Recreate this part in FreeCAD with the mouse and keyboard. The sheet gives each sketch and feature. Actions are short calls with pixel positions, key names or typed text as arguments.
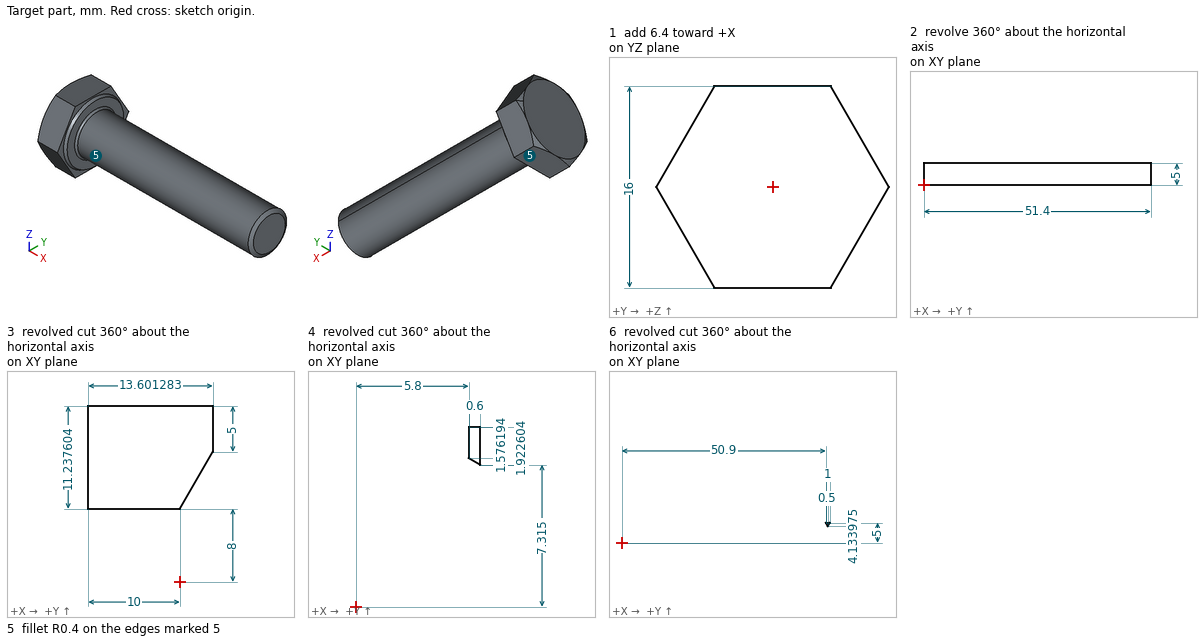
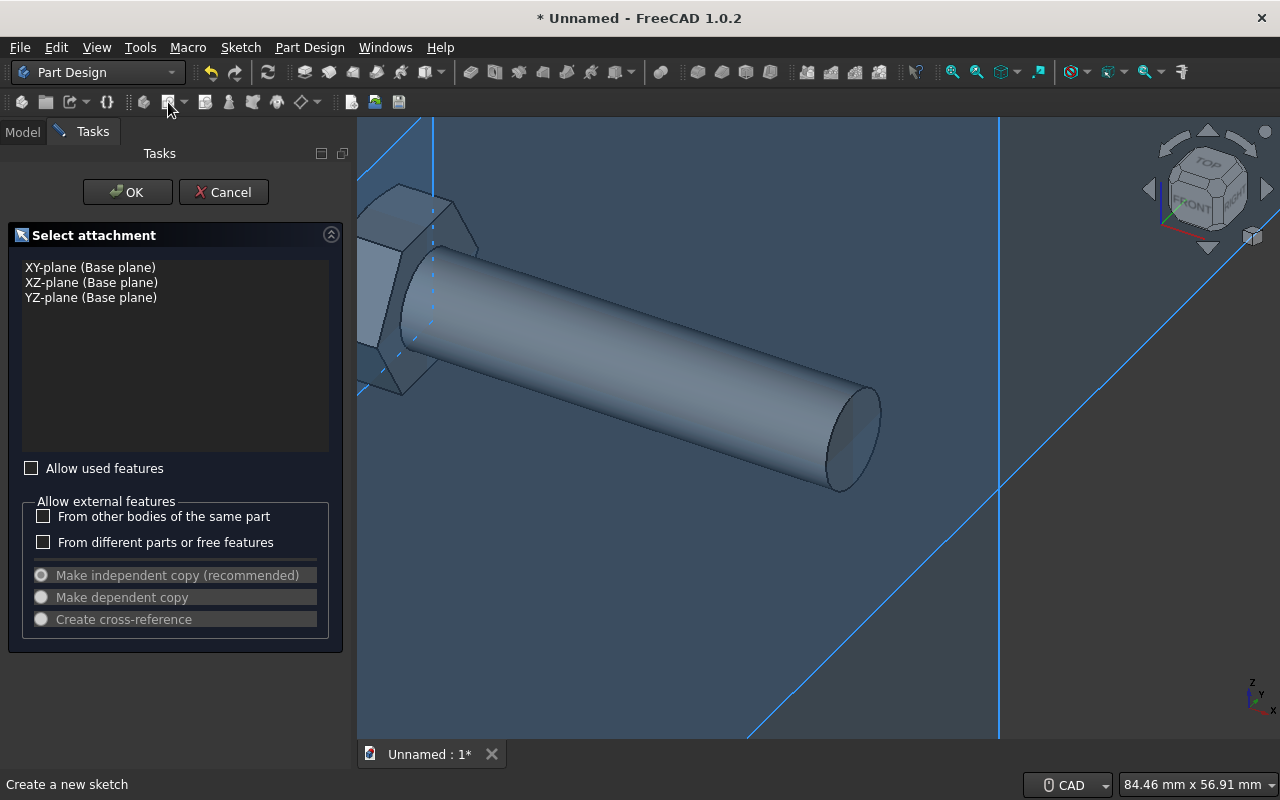
click(82, 268)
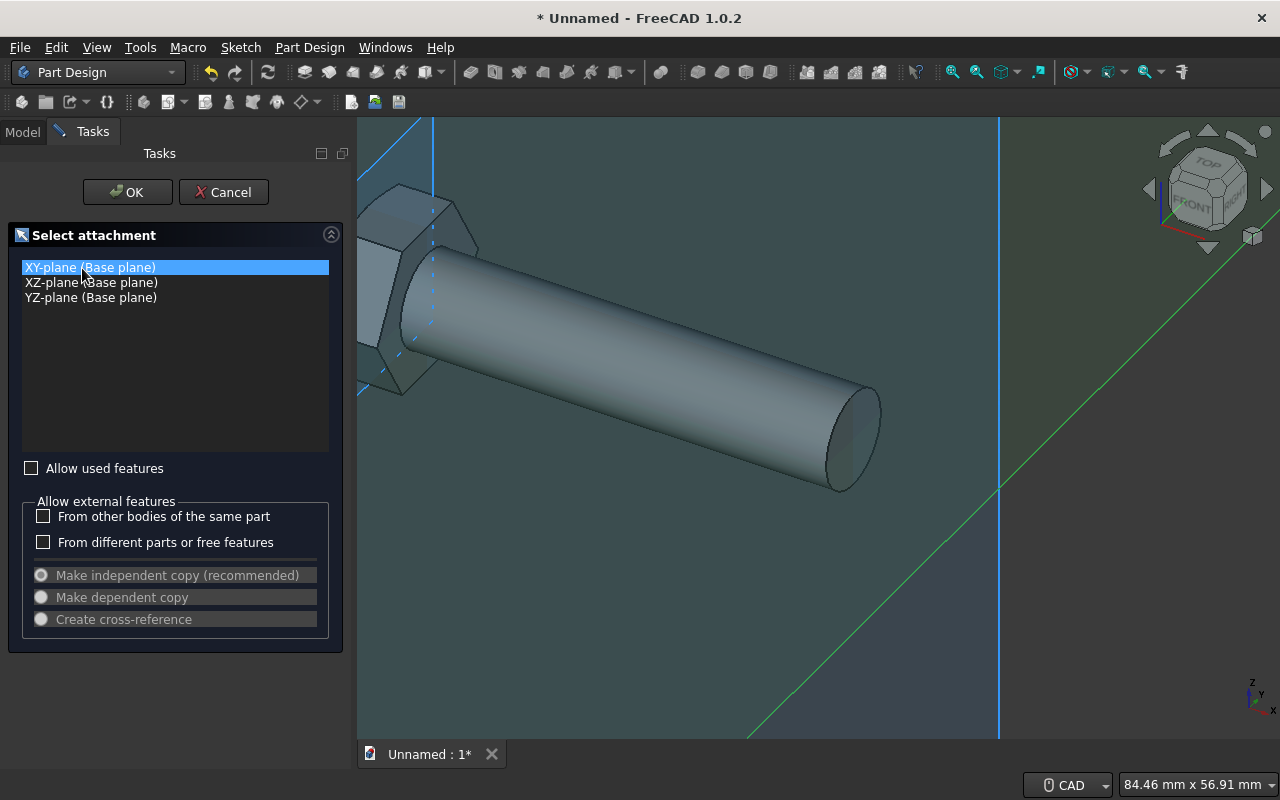
click(128, 192)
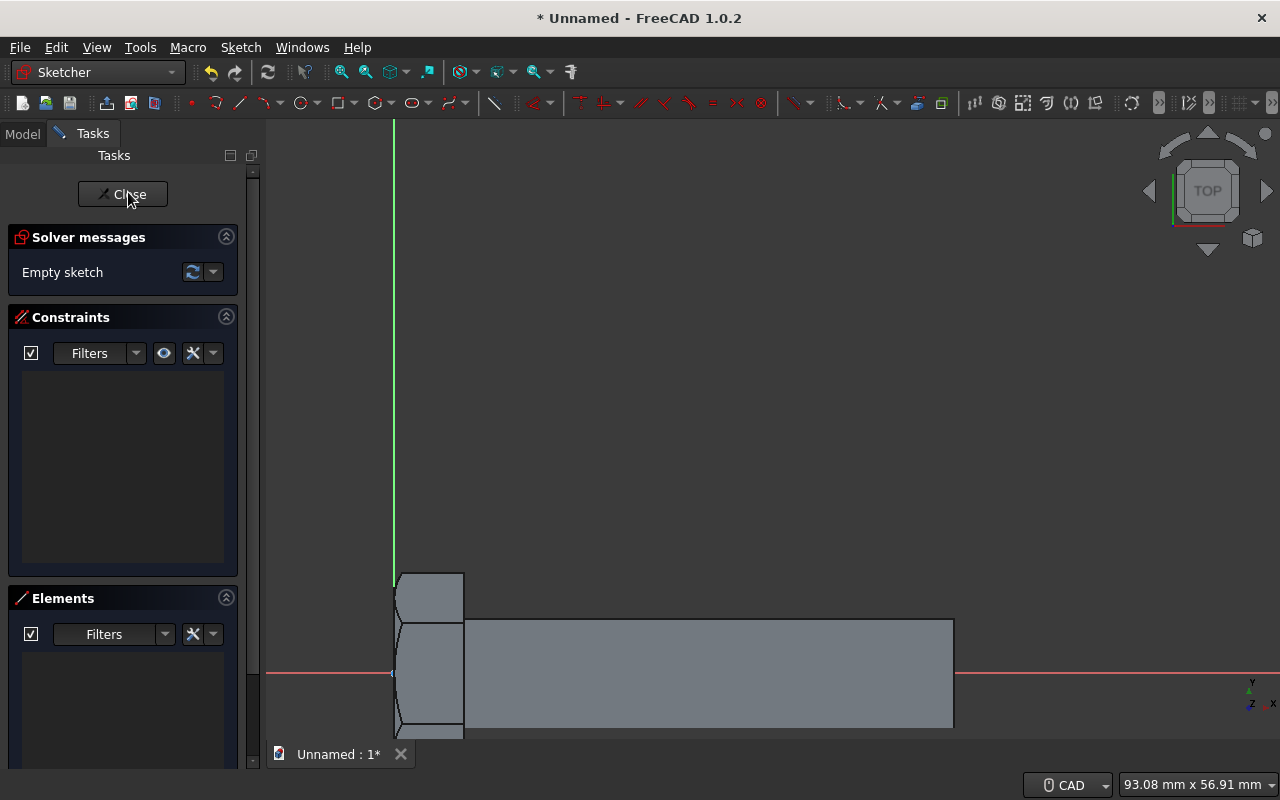
click(156, 104)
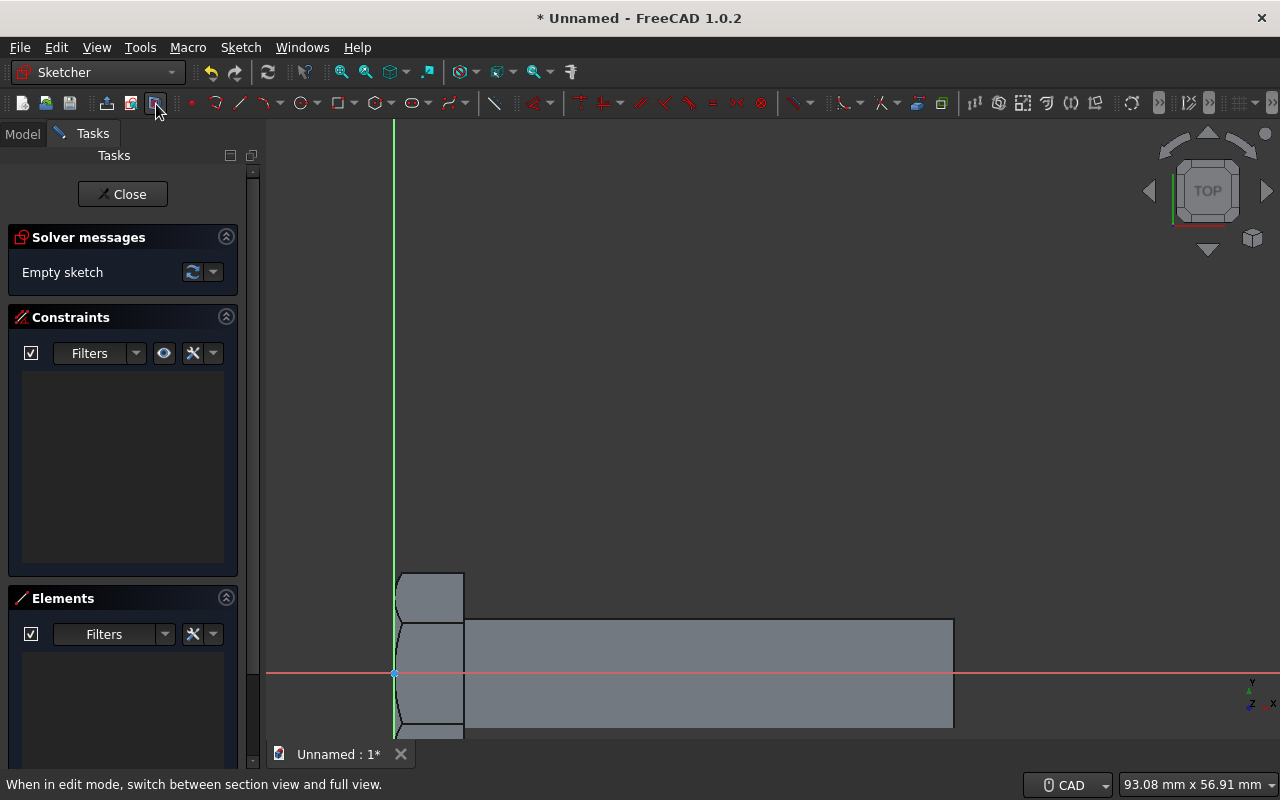
scroll(448, 591, up, 15)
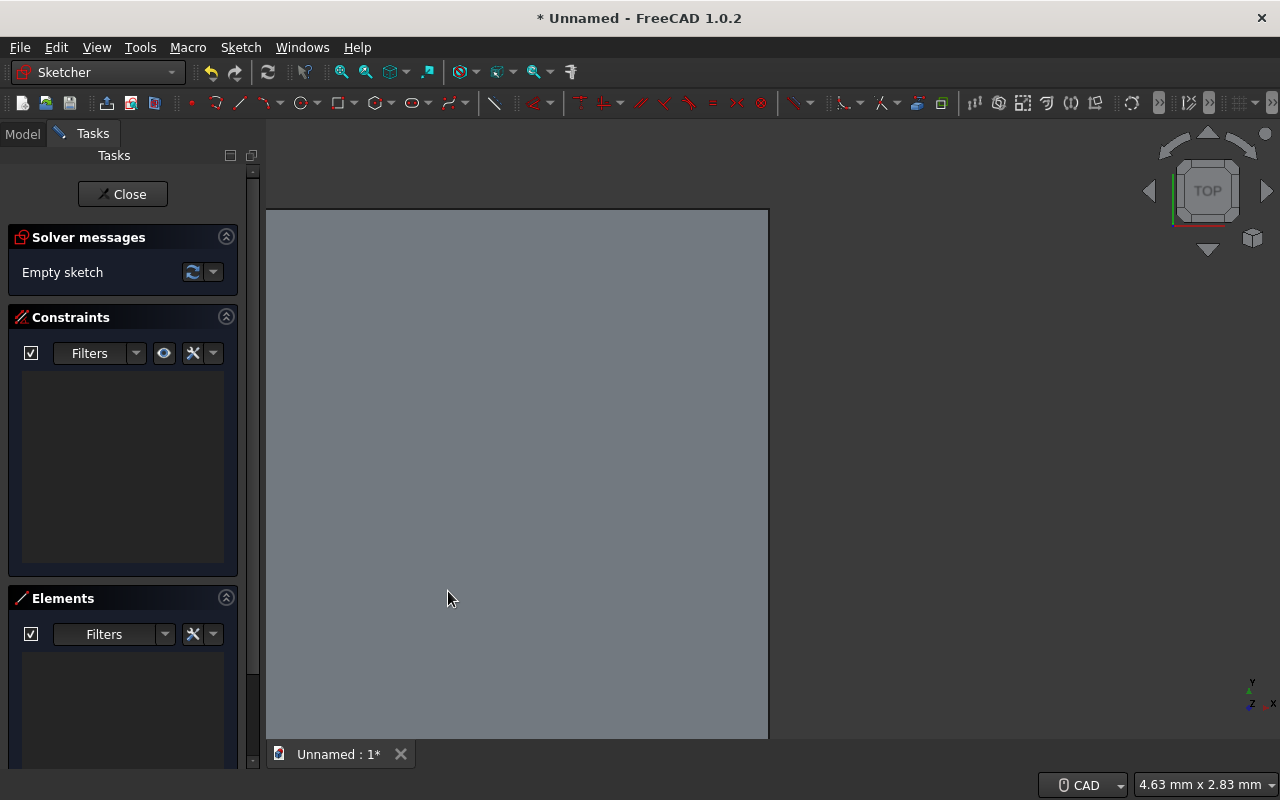
click(216, 104)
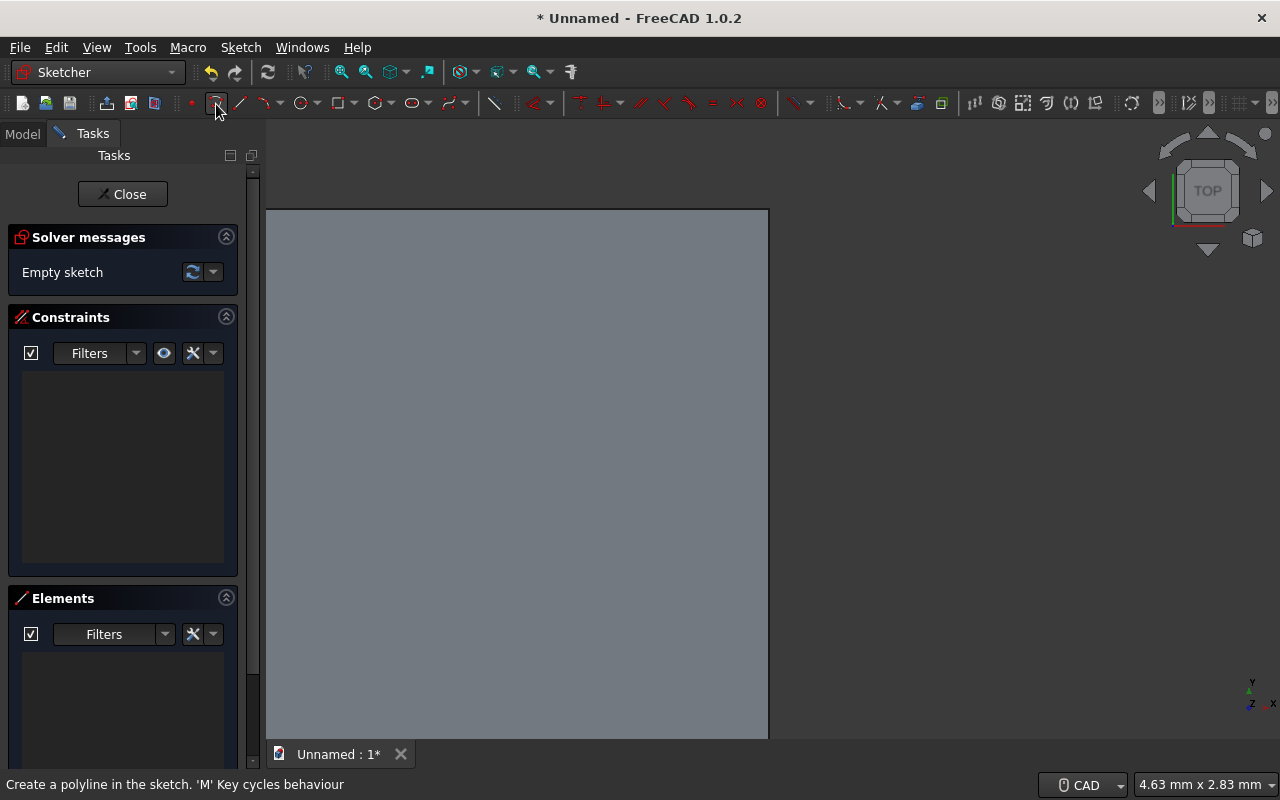
click(637, 554)
click(769, 630)
click(769, 209)
click(637, 209)
click(637, 555)
key(Escape)
key(Escape)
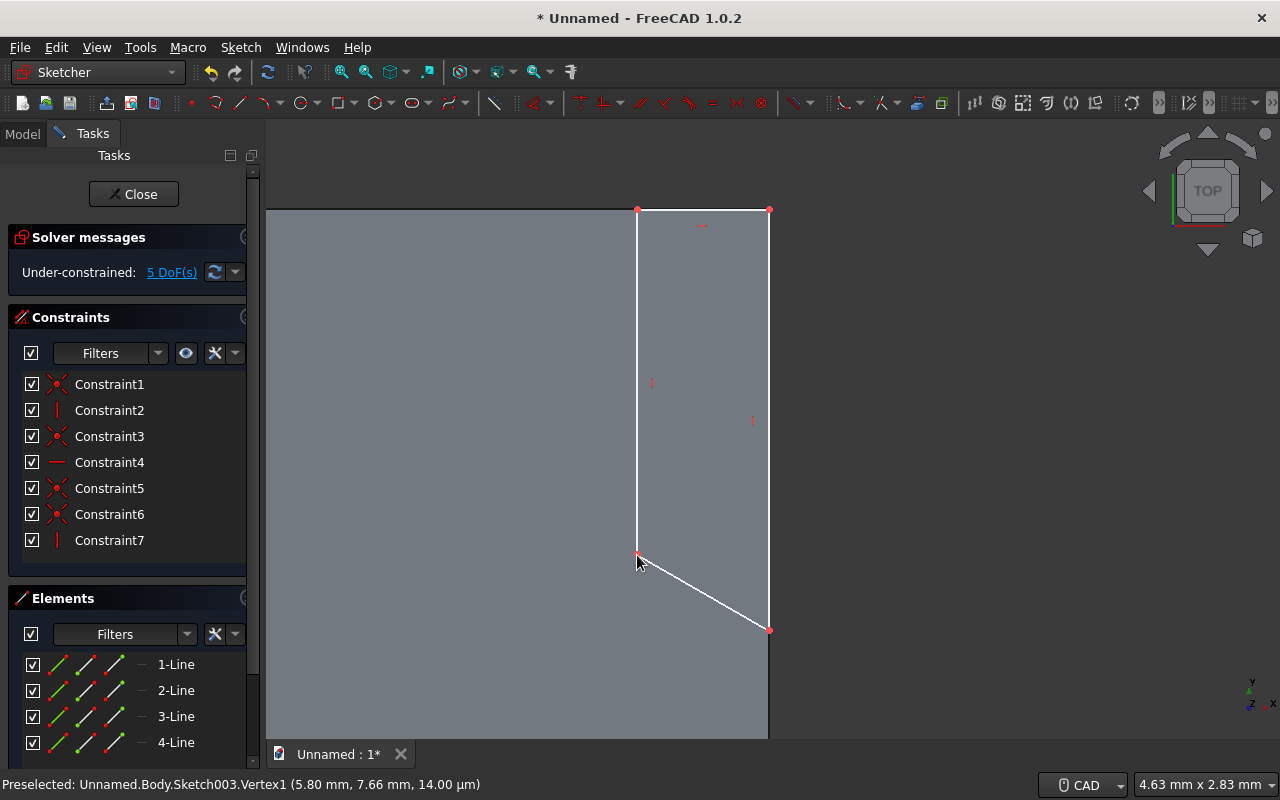
click(534, 104)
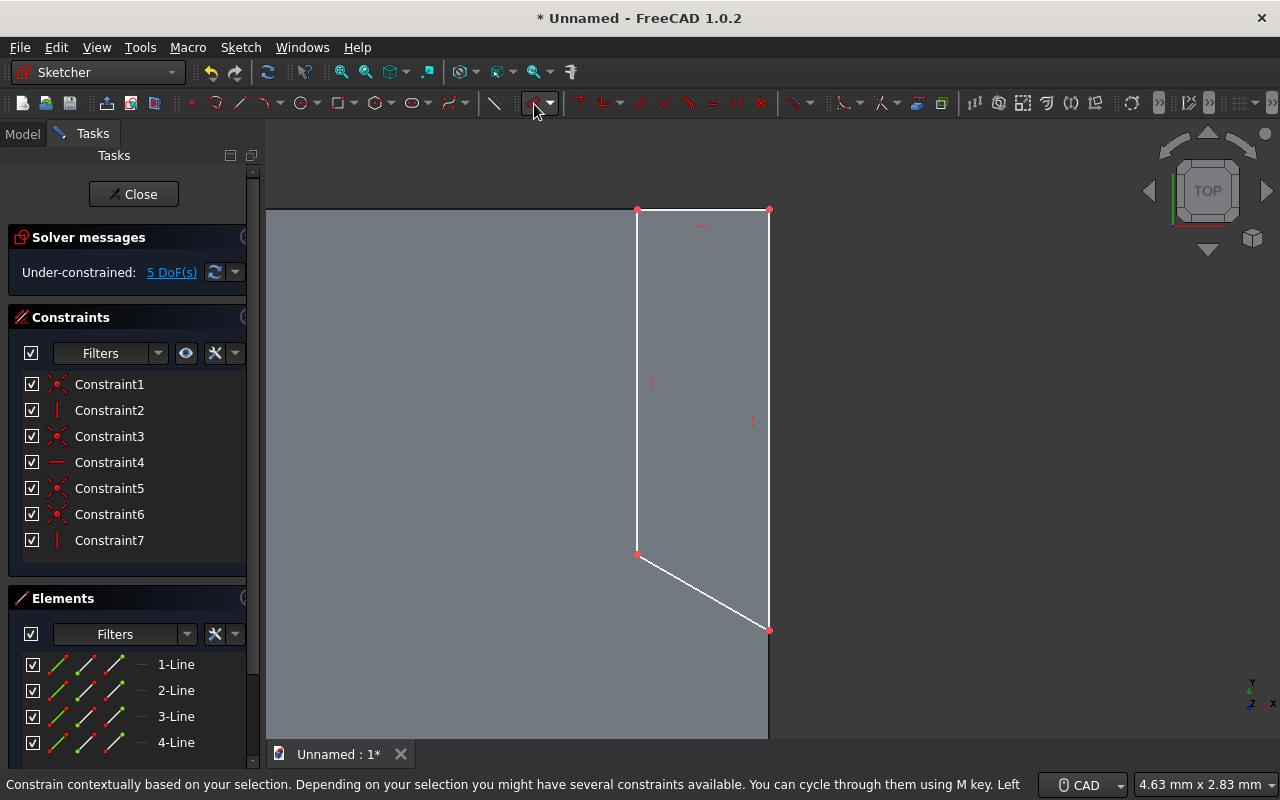
click(729, 210)
click(703, 176)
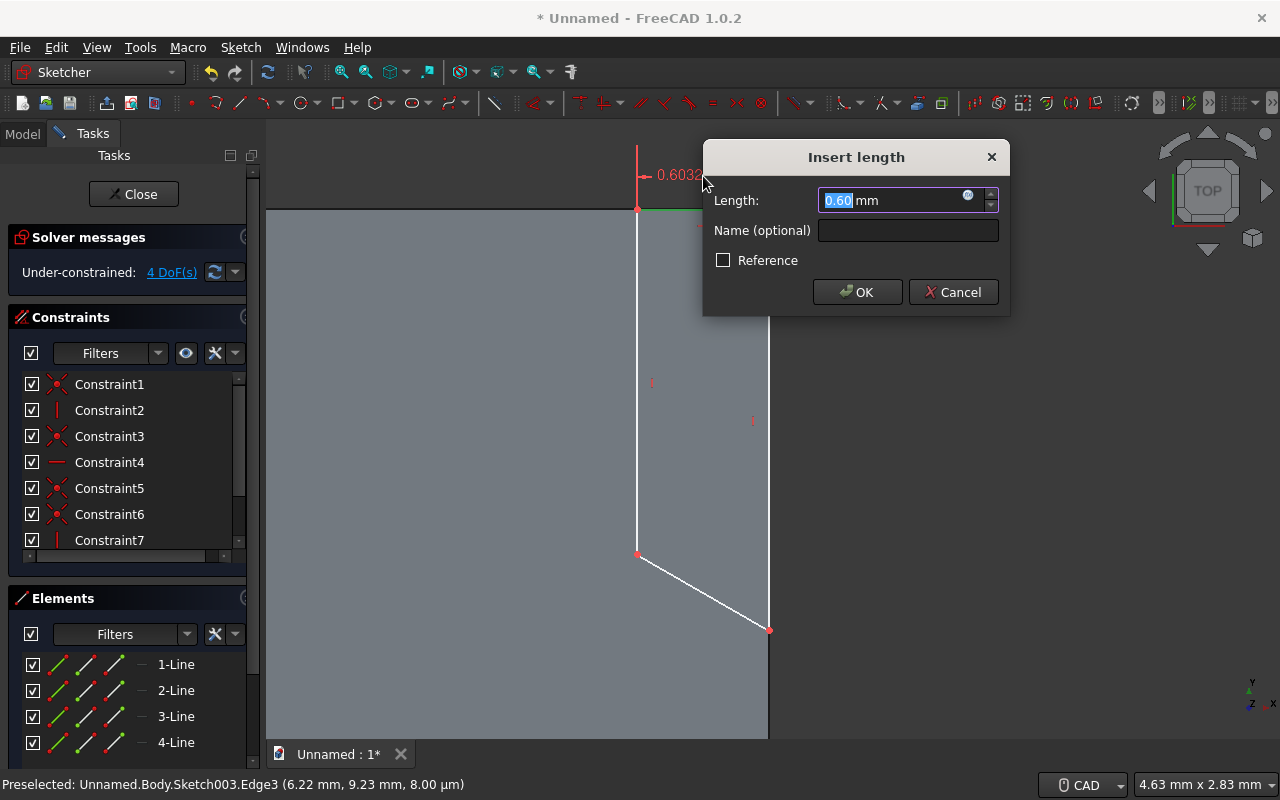
text(0.6)
key(Return)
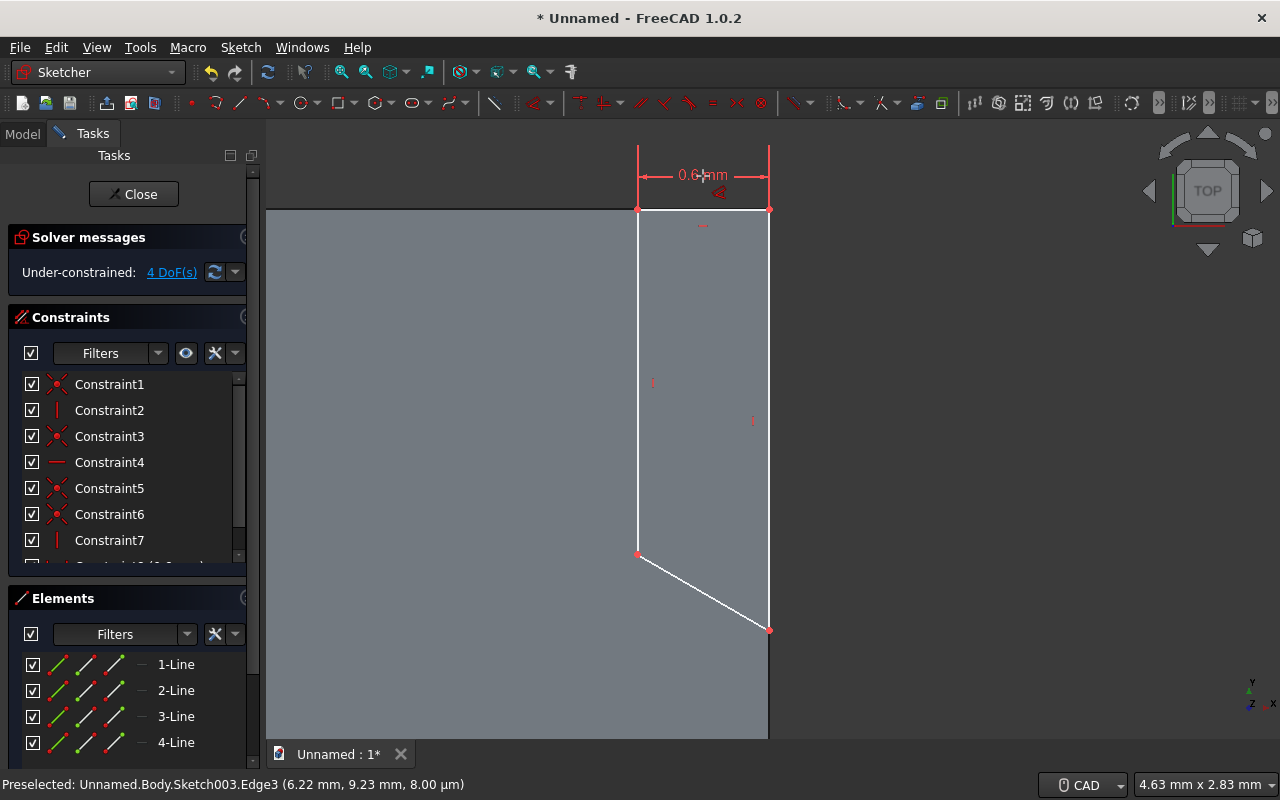
click(638, 555)
click(466, 521)